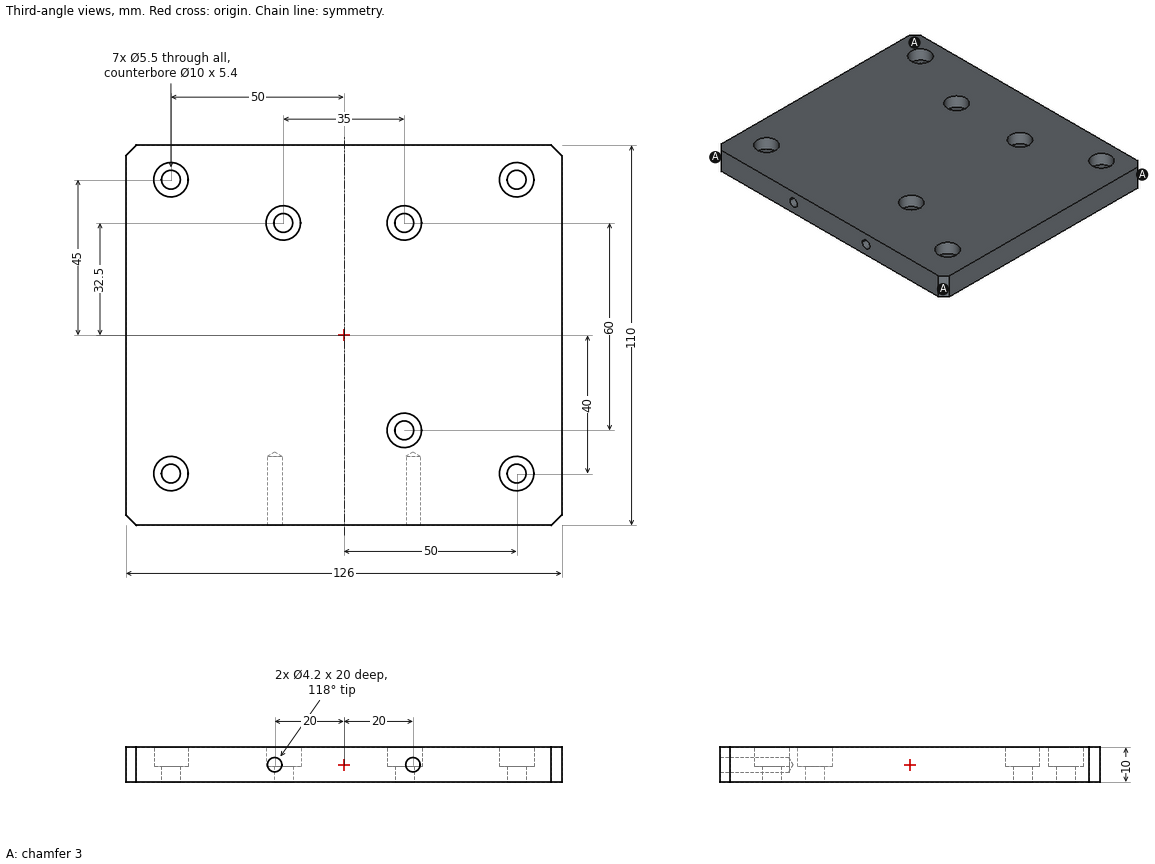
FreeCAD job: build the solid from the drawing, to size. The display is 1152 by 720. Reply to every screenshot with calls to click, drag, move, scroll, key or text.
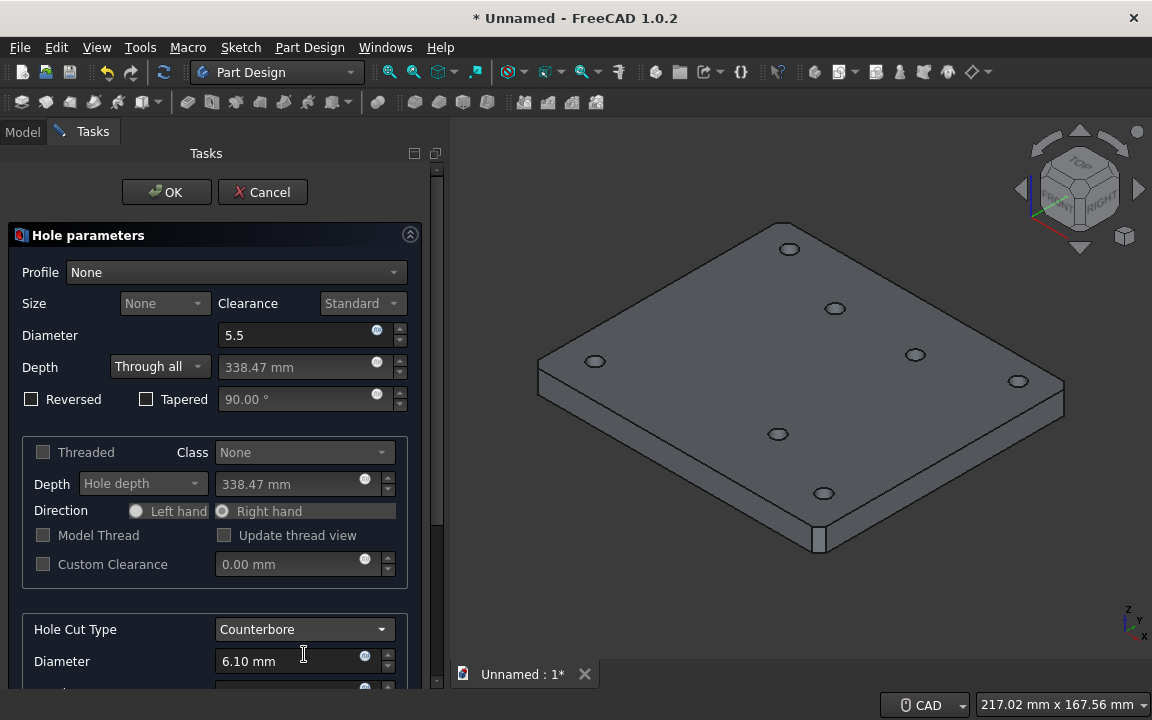
triple_click(298, 661)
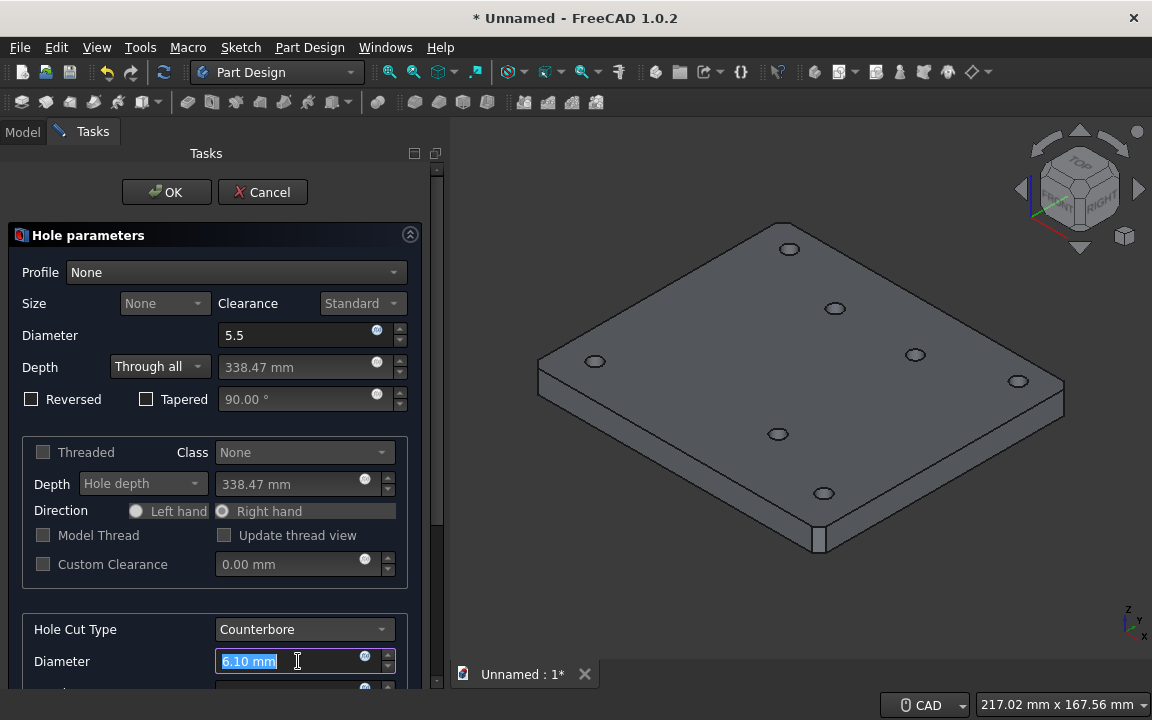
text(10)
key(Tab)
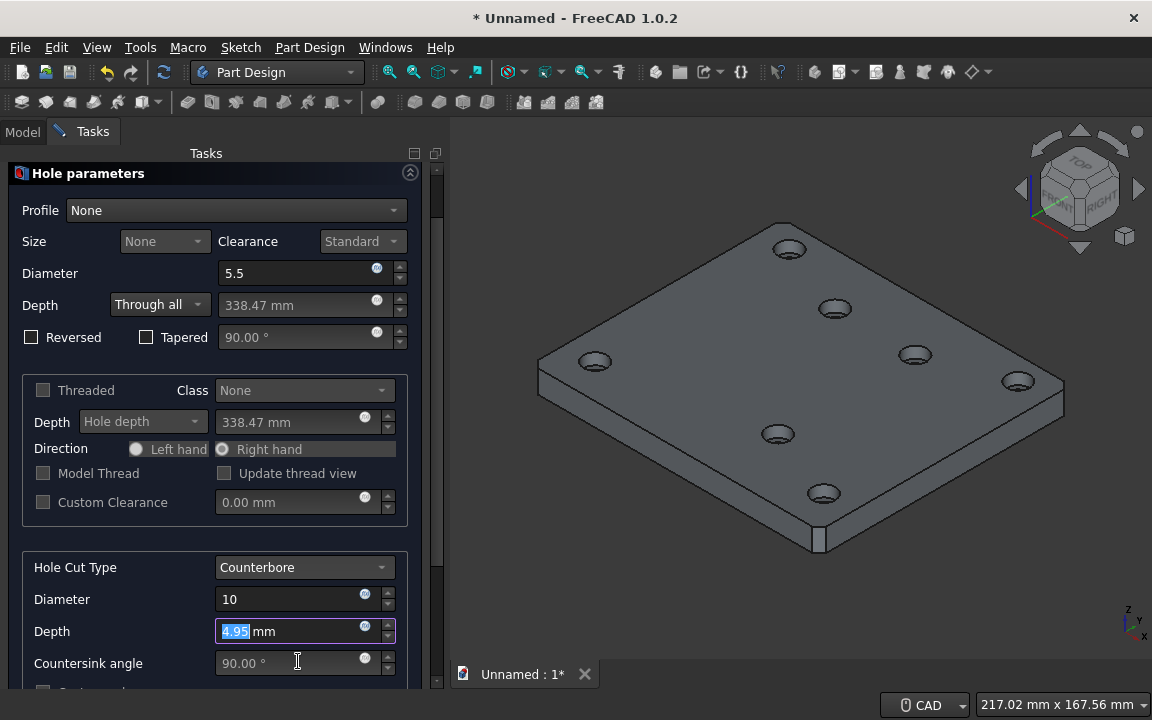
text(5.4)
key(Tab)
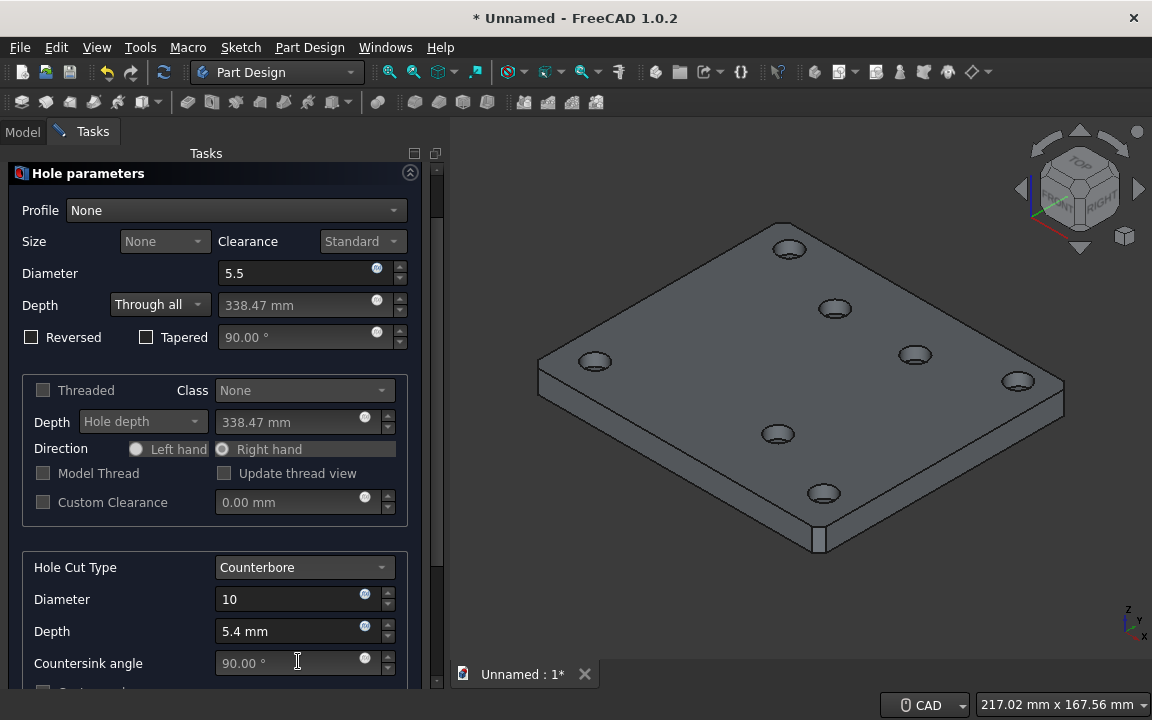
scroll(437, 426, up, 2)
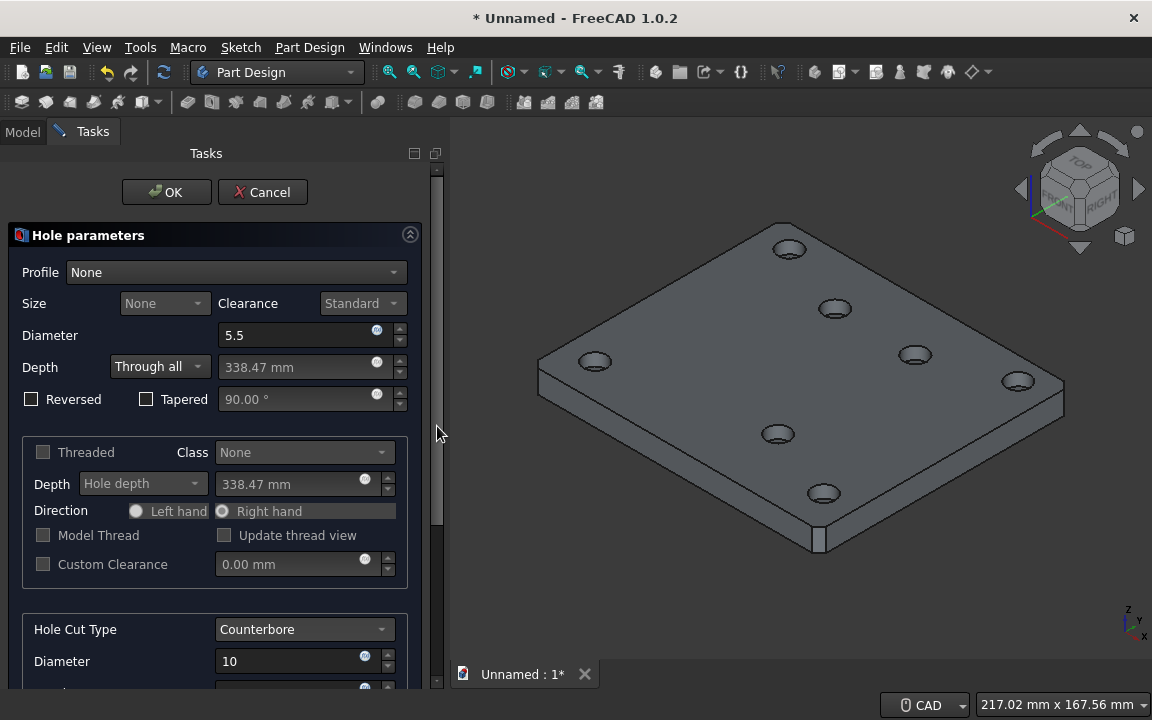
click(167, 192)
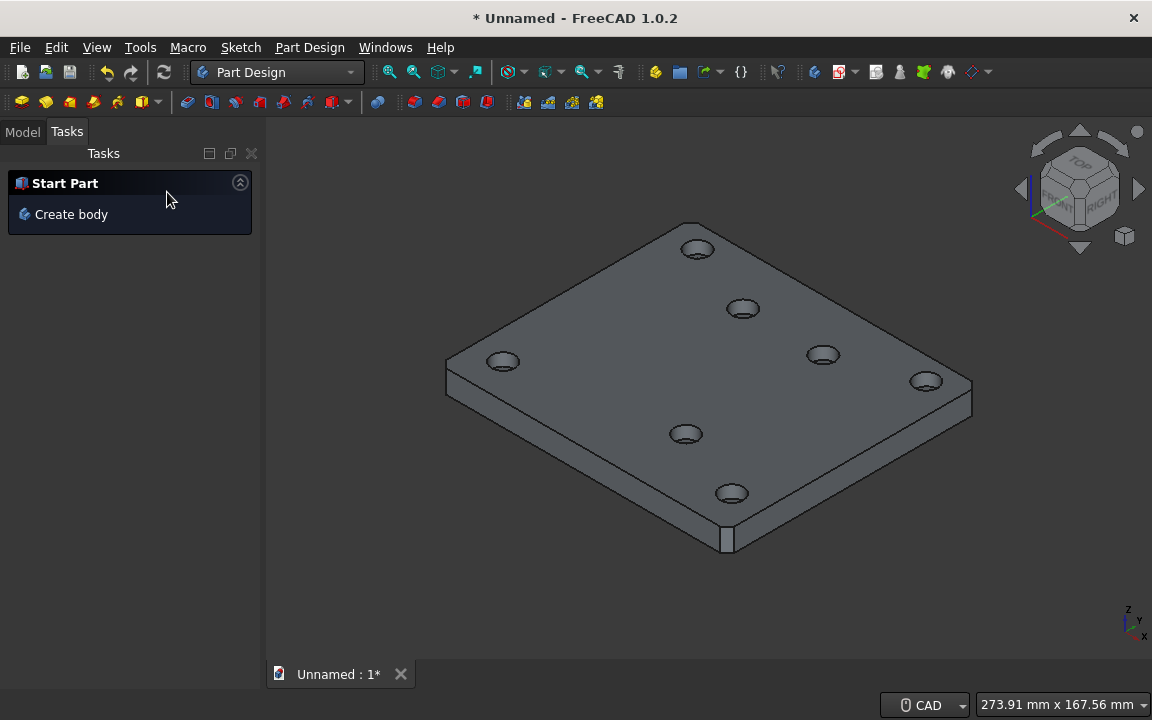
click(701, 528)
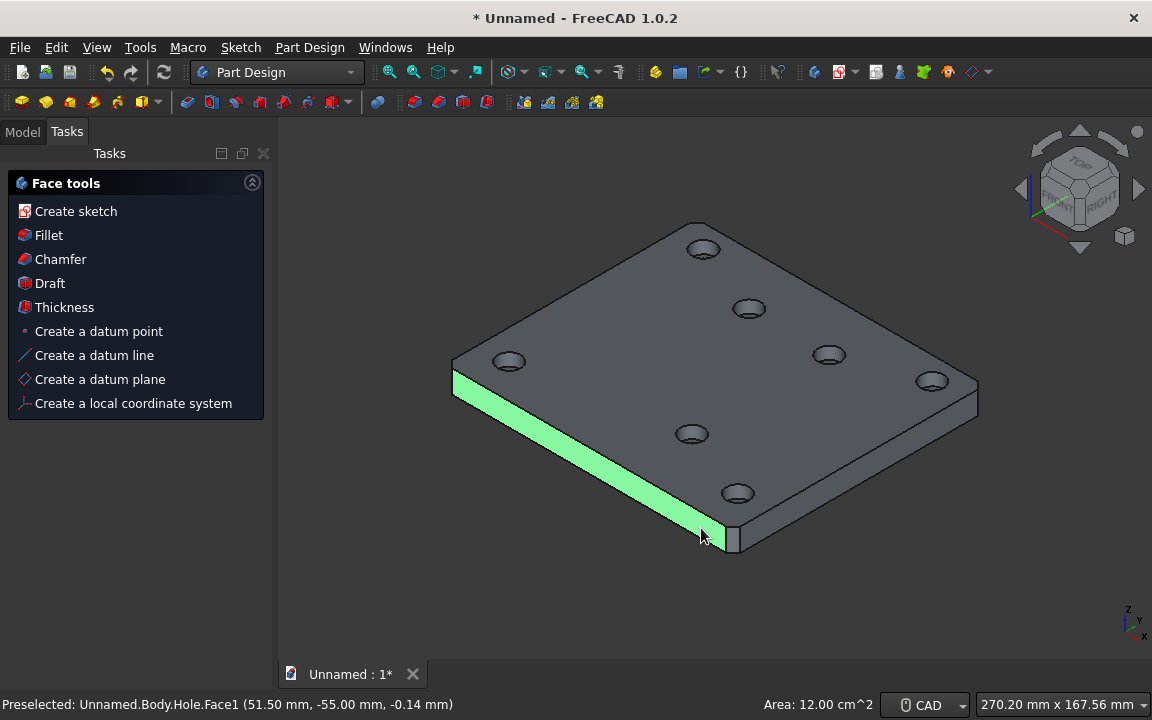
click(840, 72)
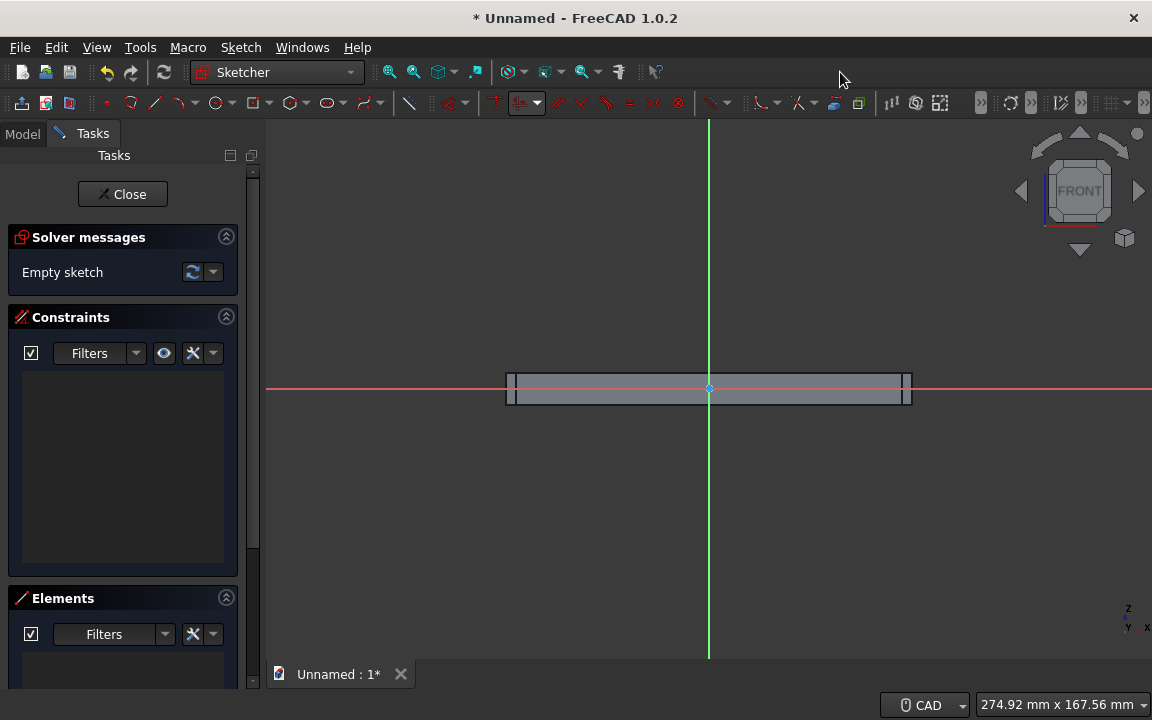
scroll(739, 389, up, 6)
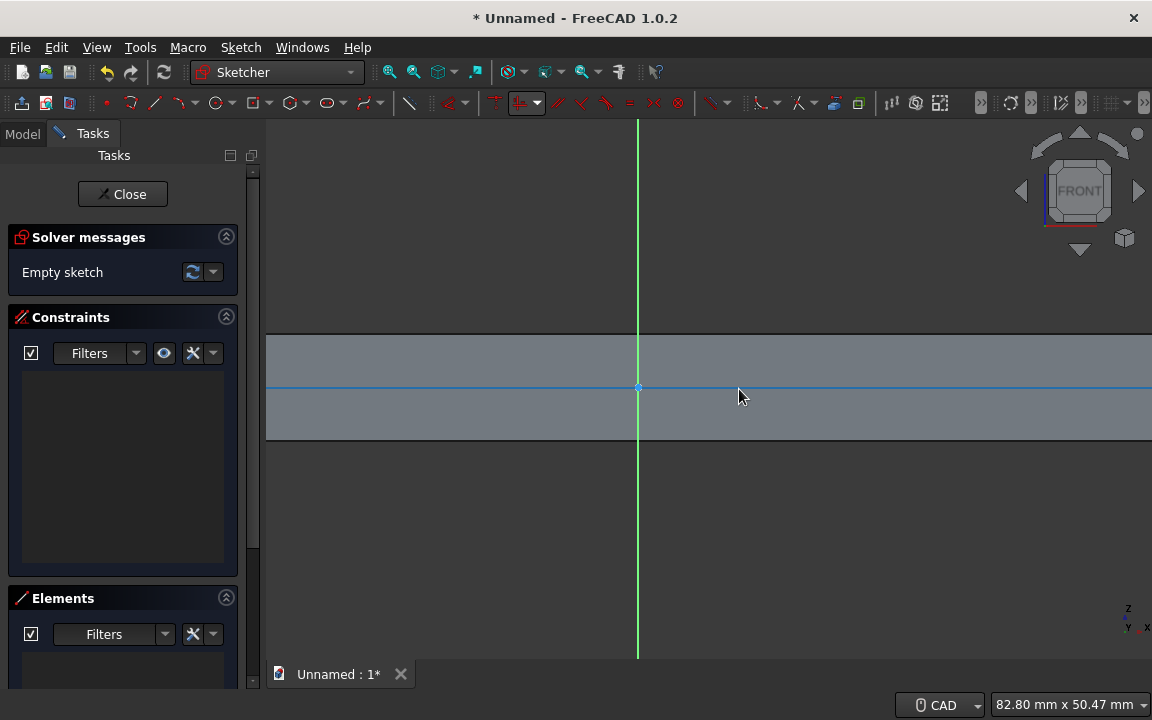
click(216, 104)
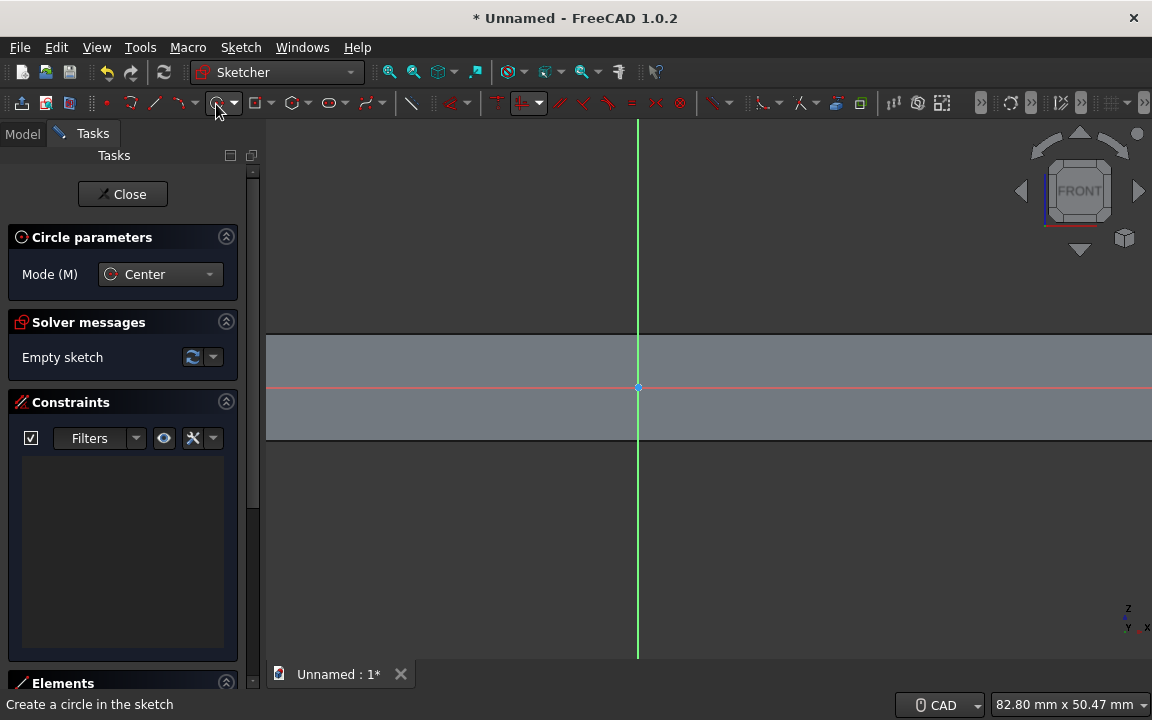
click(424, 388)
move(440, 372)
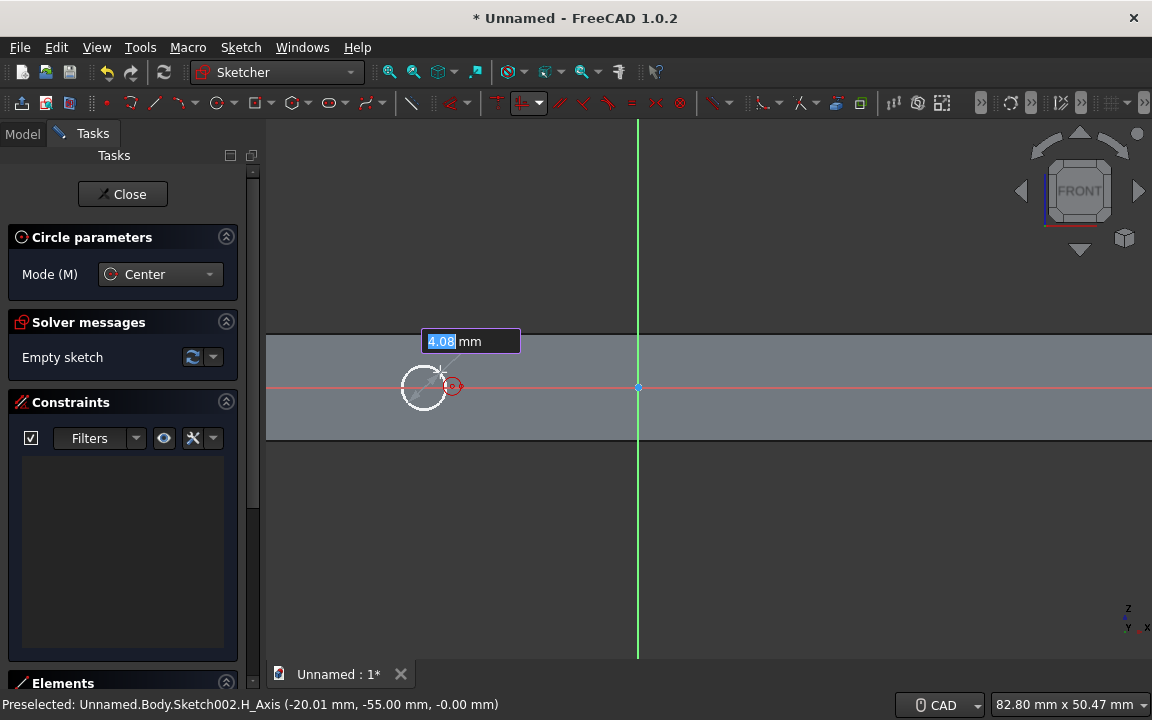
text(4.2)
key(Return)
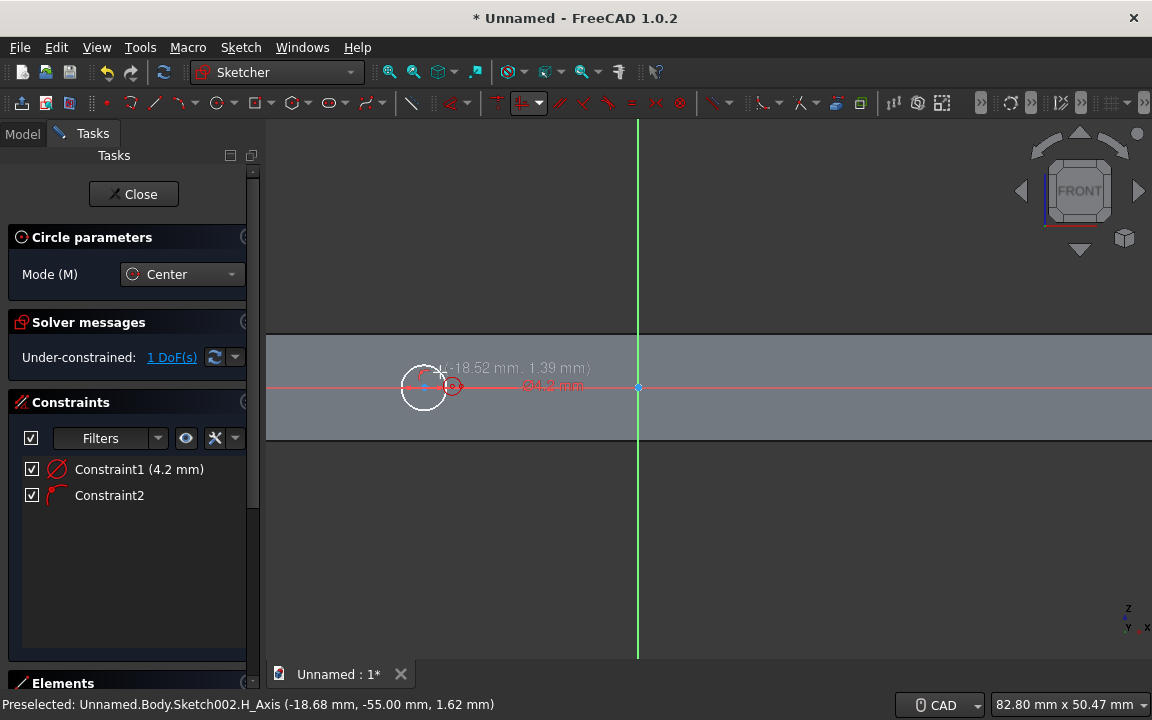
click(852, 388)
move(868, 372)